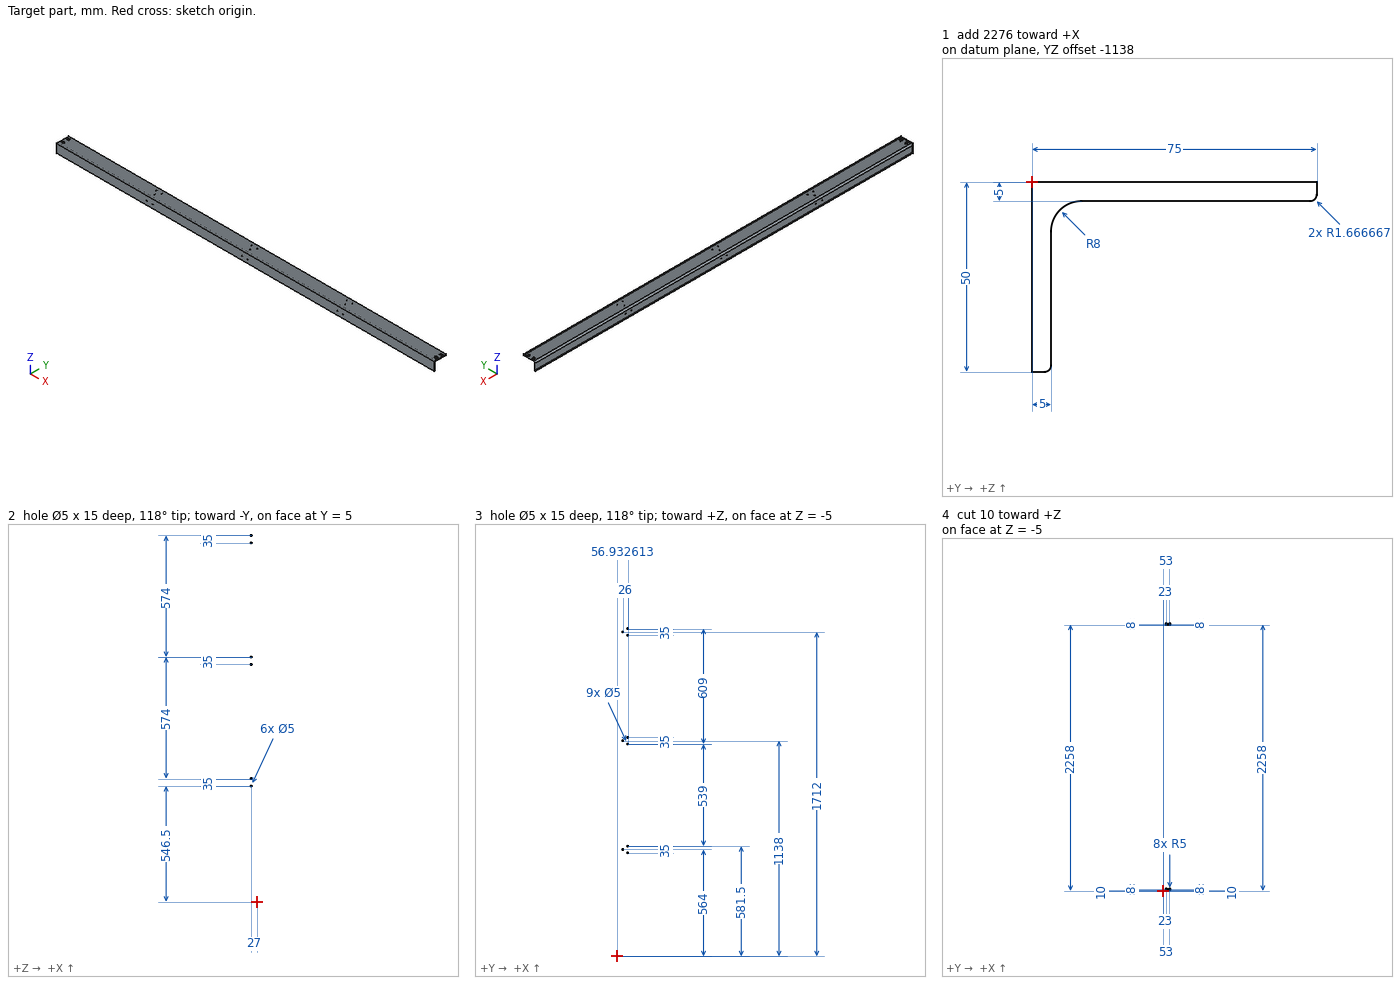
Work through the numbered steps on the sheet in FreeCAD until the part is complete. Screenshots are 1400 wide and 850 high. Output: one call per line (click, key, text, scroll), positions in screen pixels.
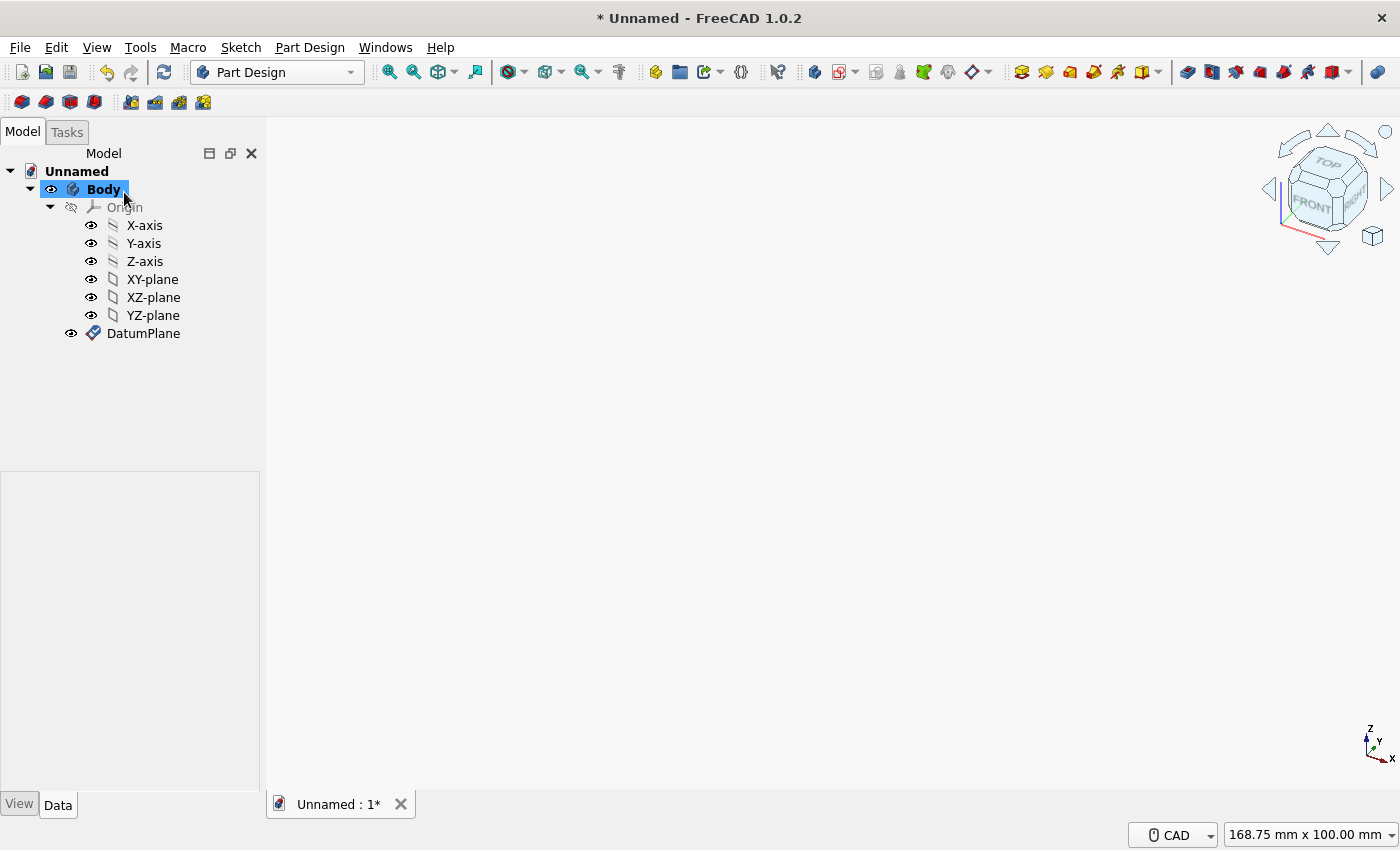
click(116, 333)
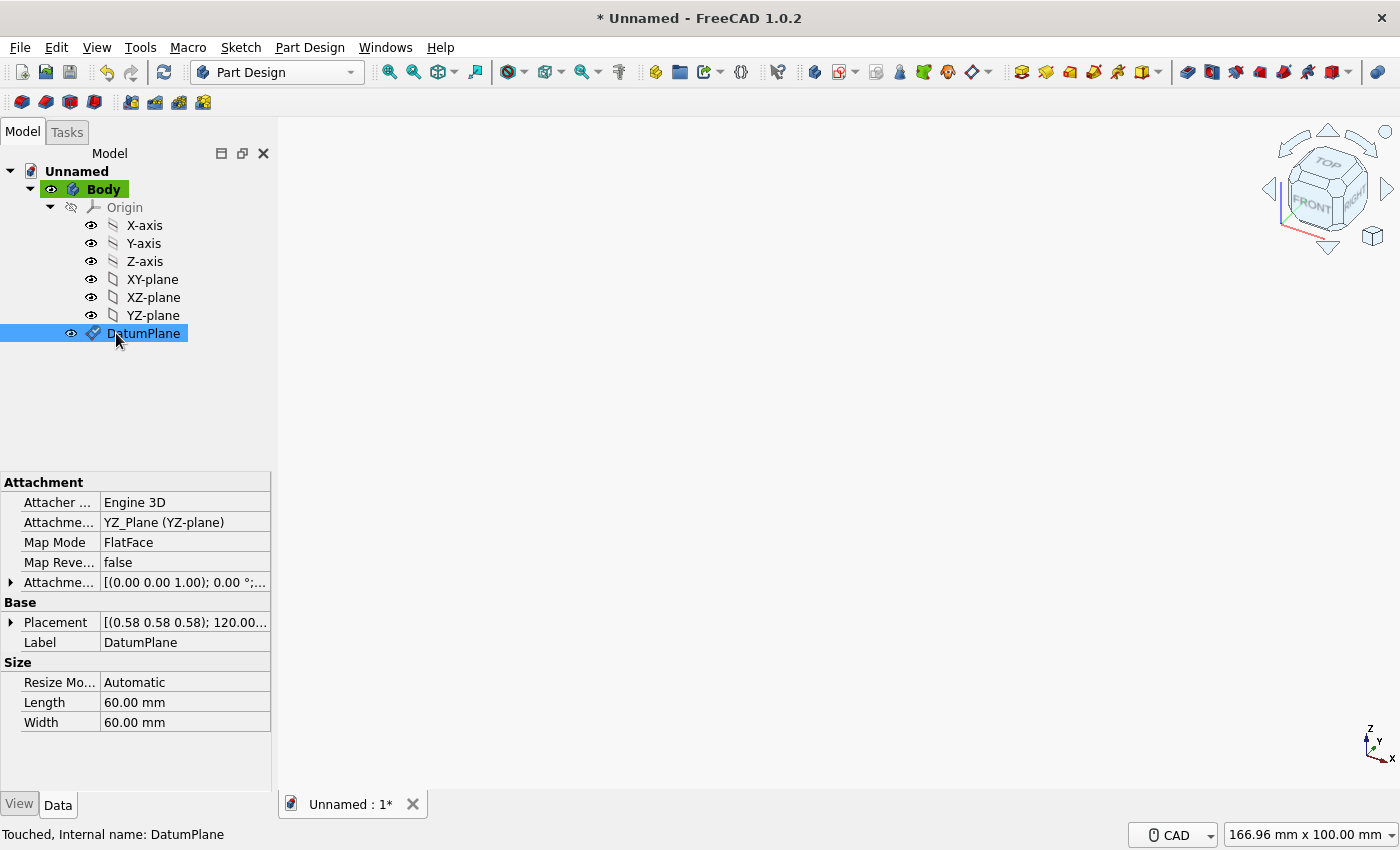
click(840, 72)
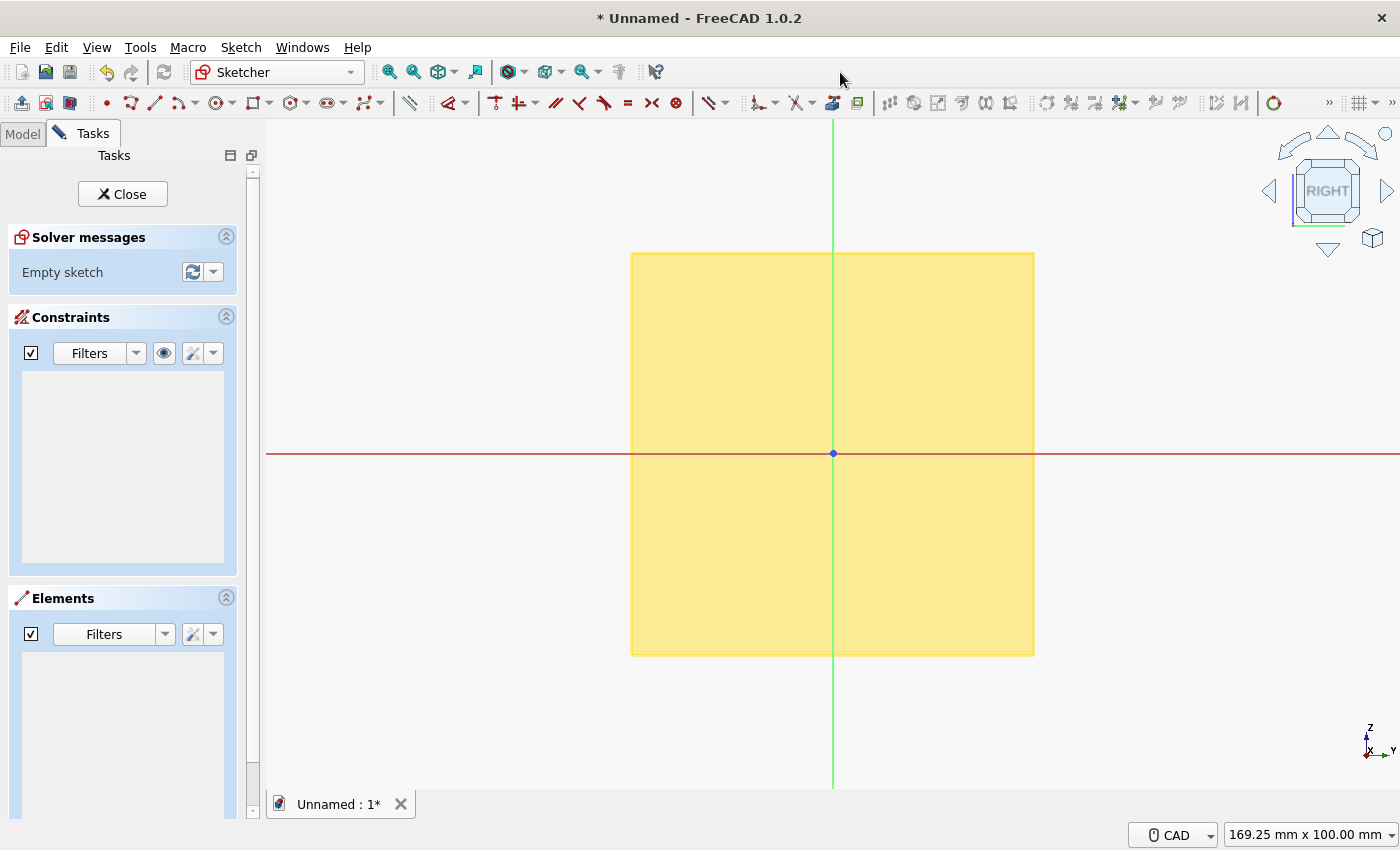
scroll(294, 147, down, 1)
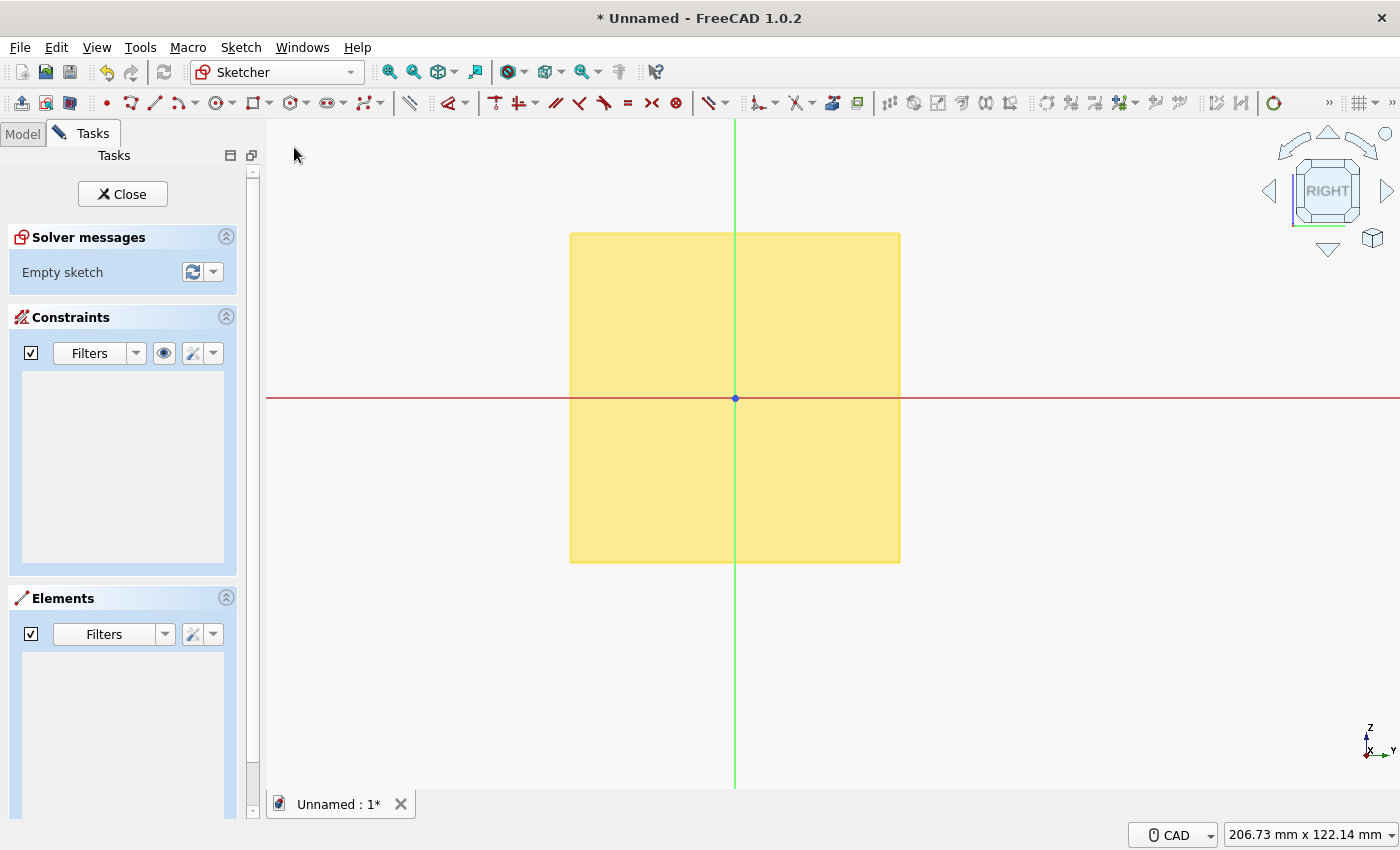
scroll(1235, 701, up, 2)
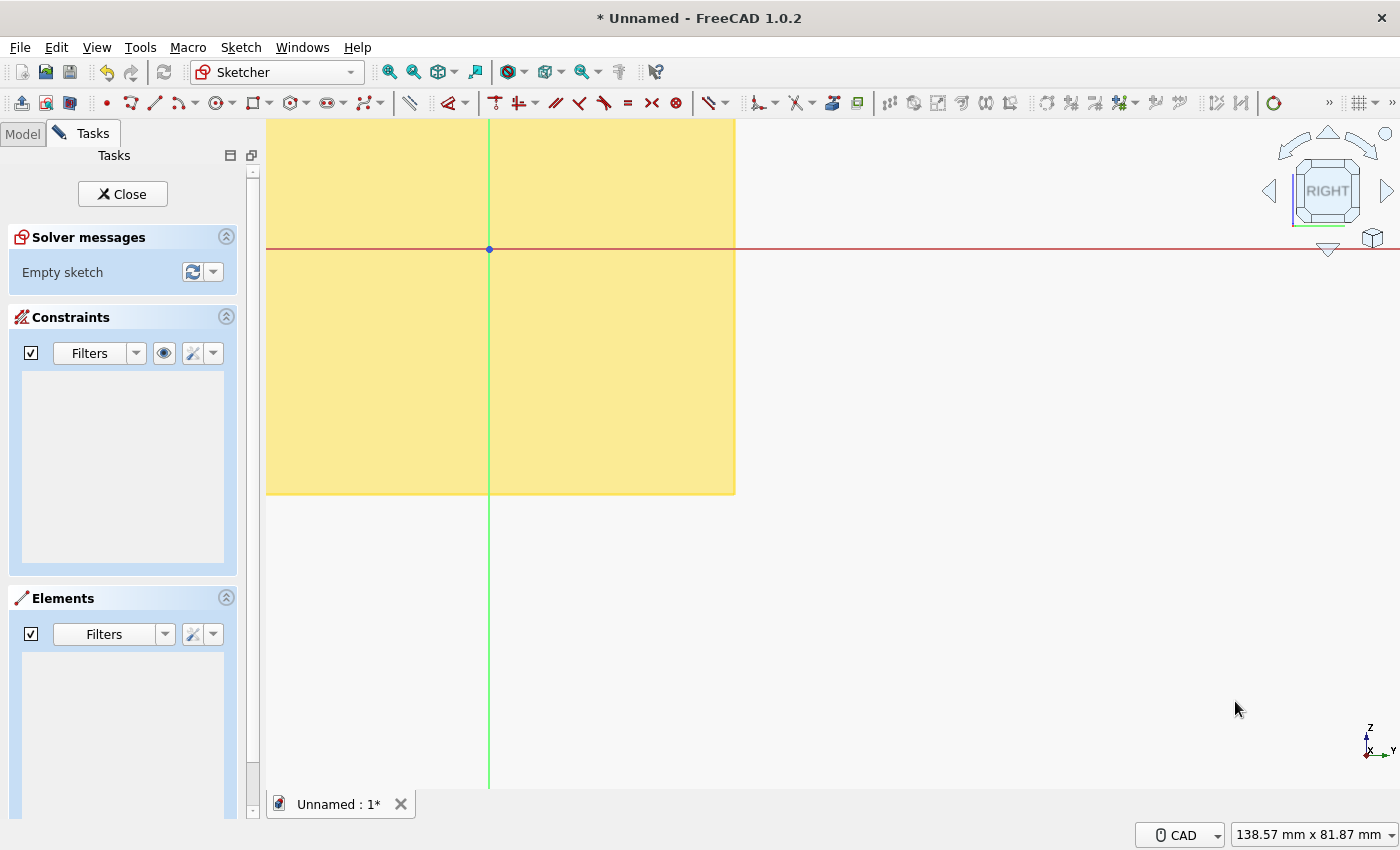
click(156, 104)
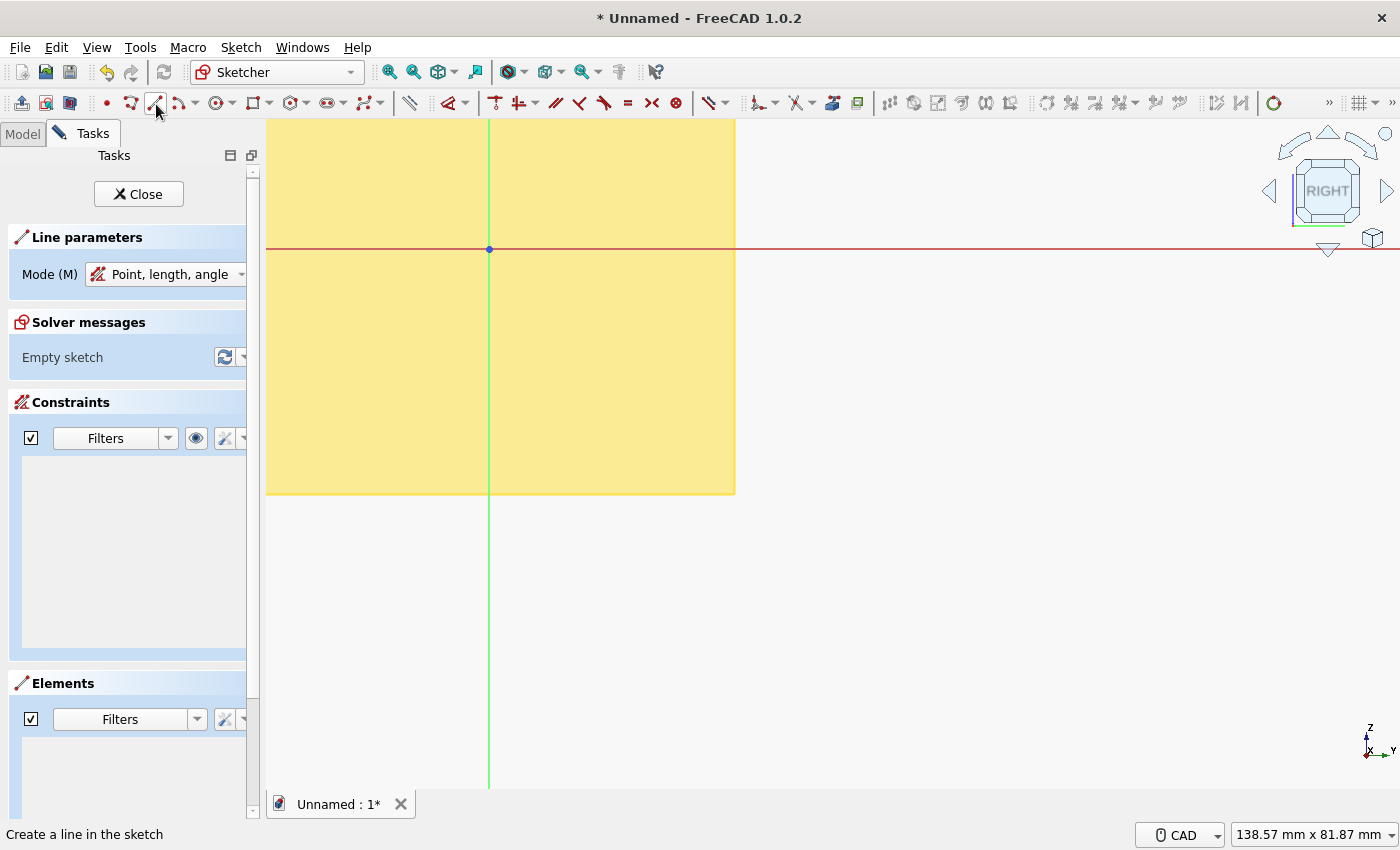
click(530, 645)
click(530, 355)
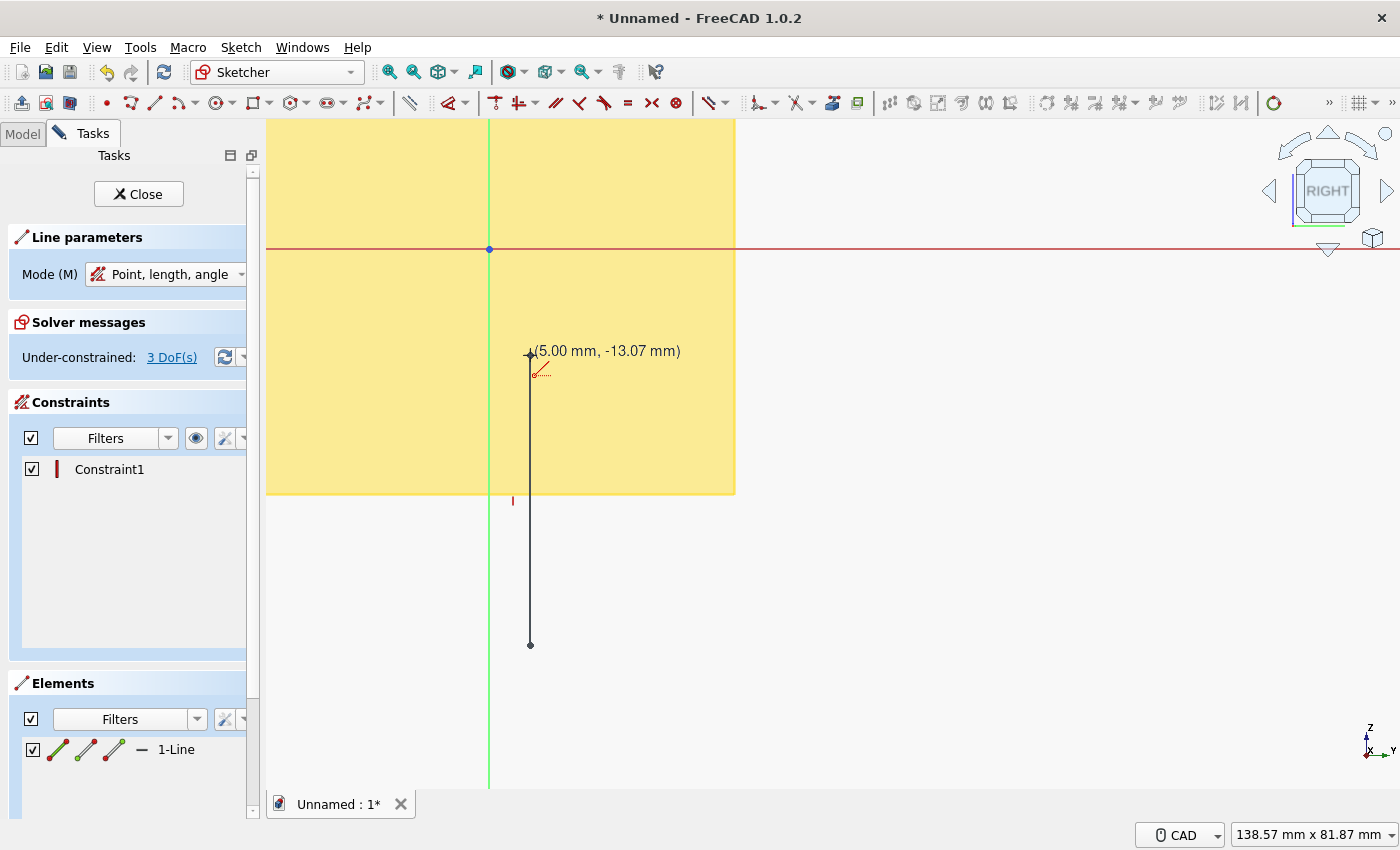
click(595, 290)
click(1089, 290)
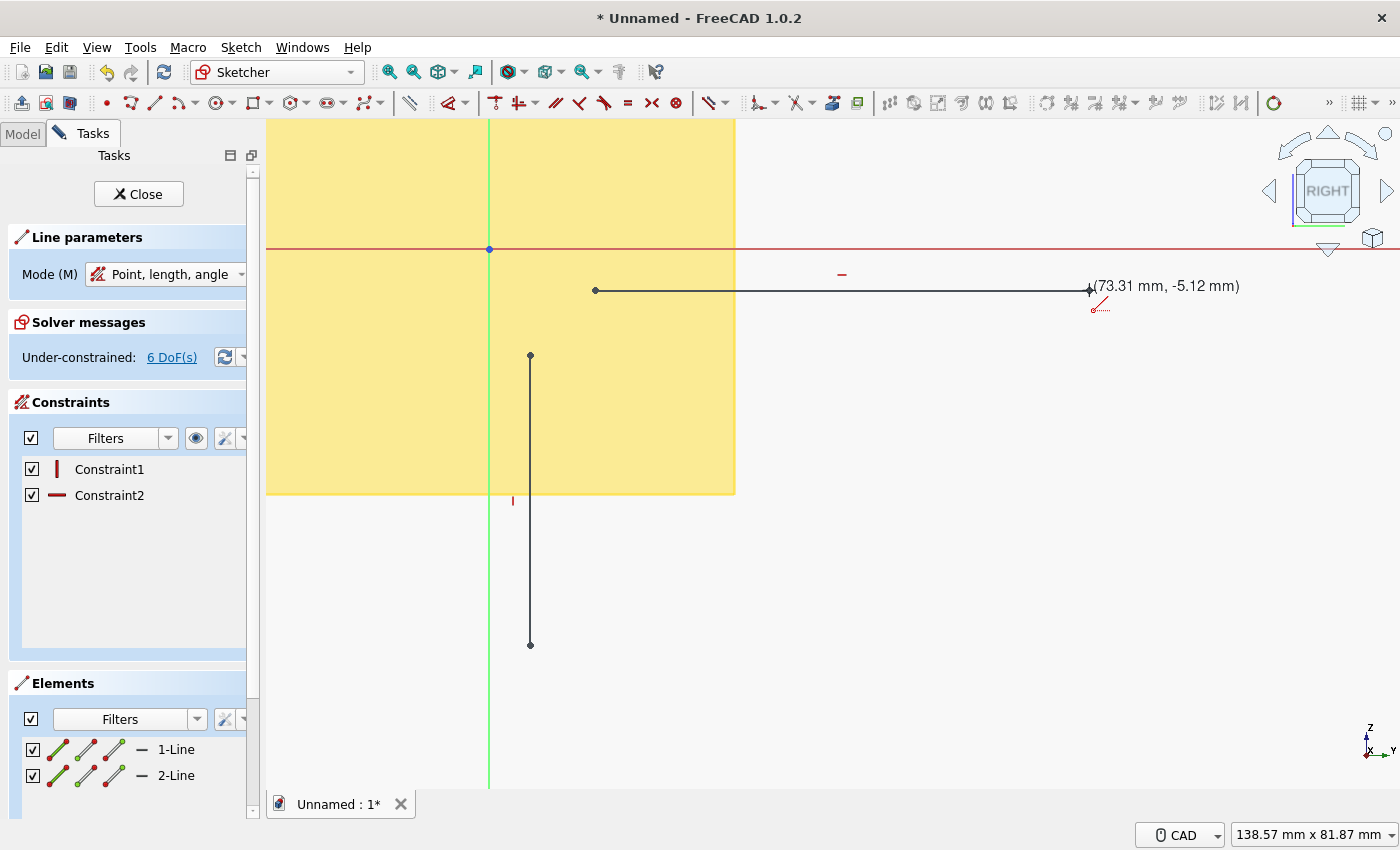
click(132, 104)